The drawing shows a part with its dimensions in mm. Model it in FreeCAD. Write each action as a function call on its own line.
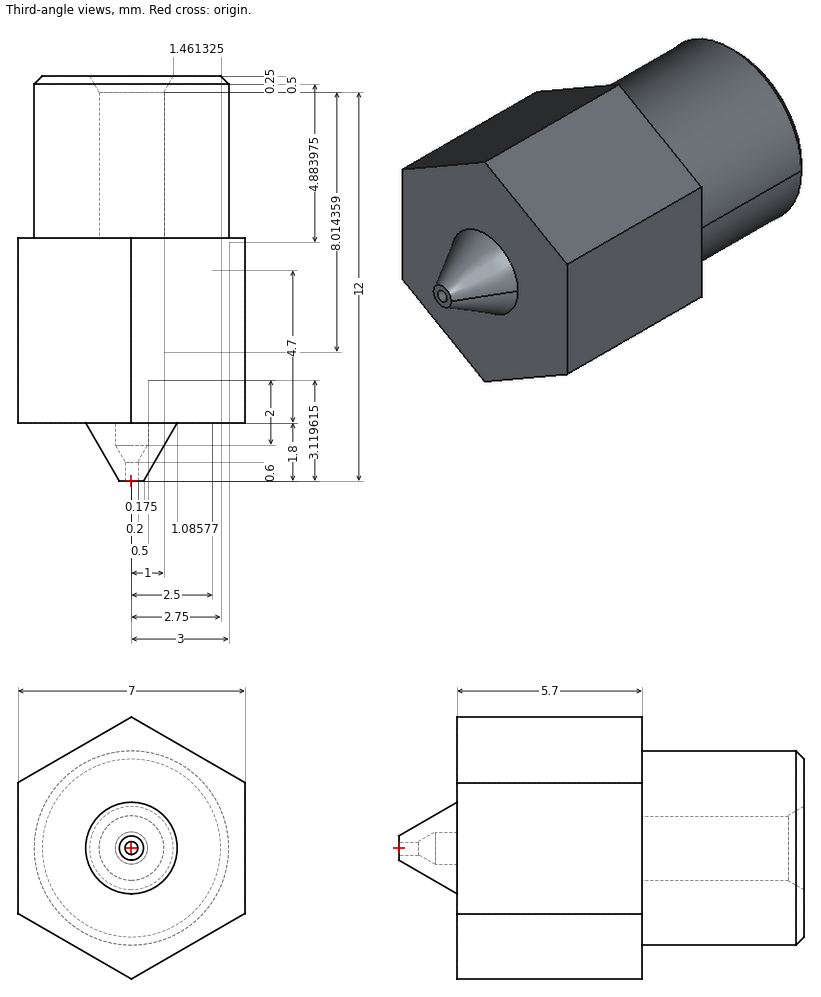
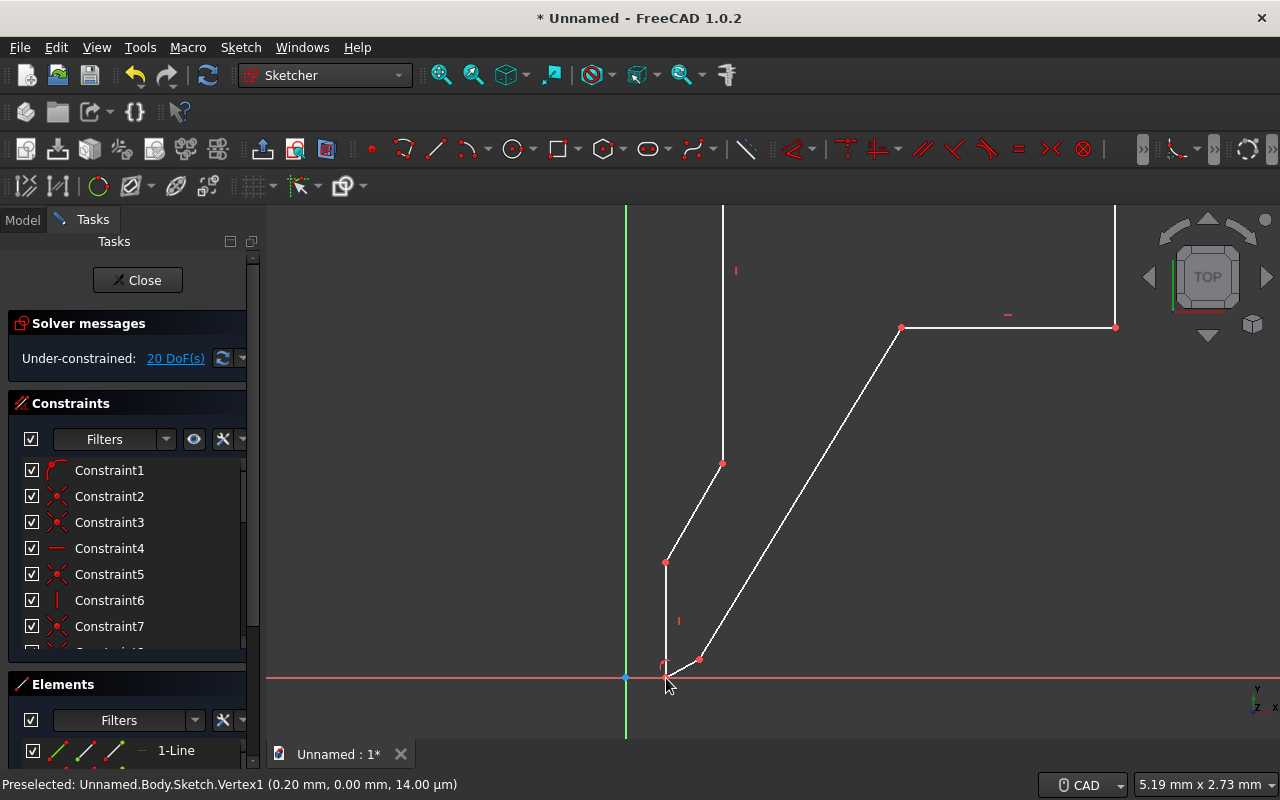
click(689, 665)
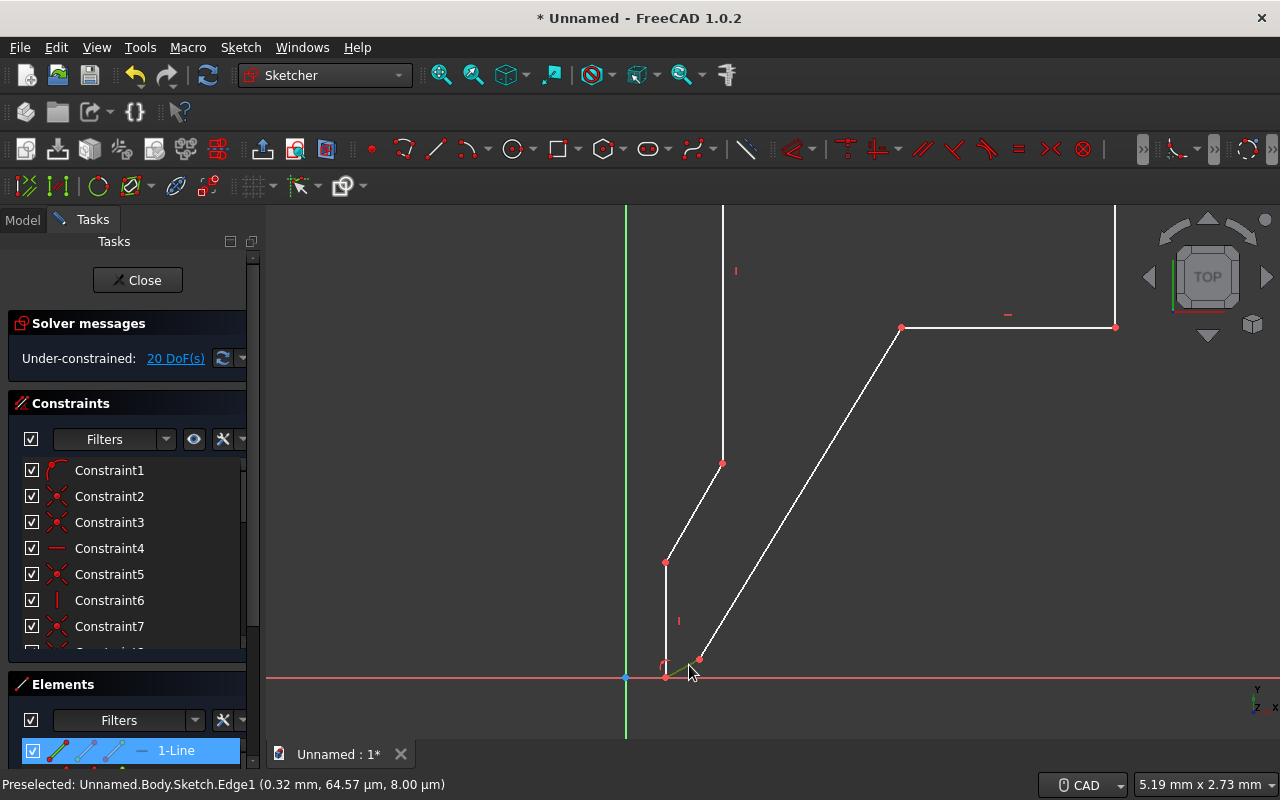
click(900, 150)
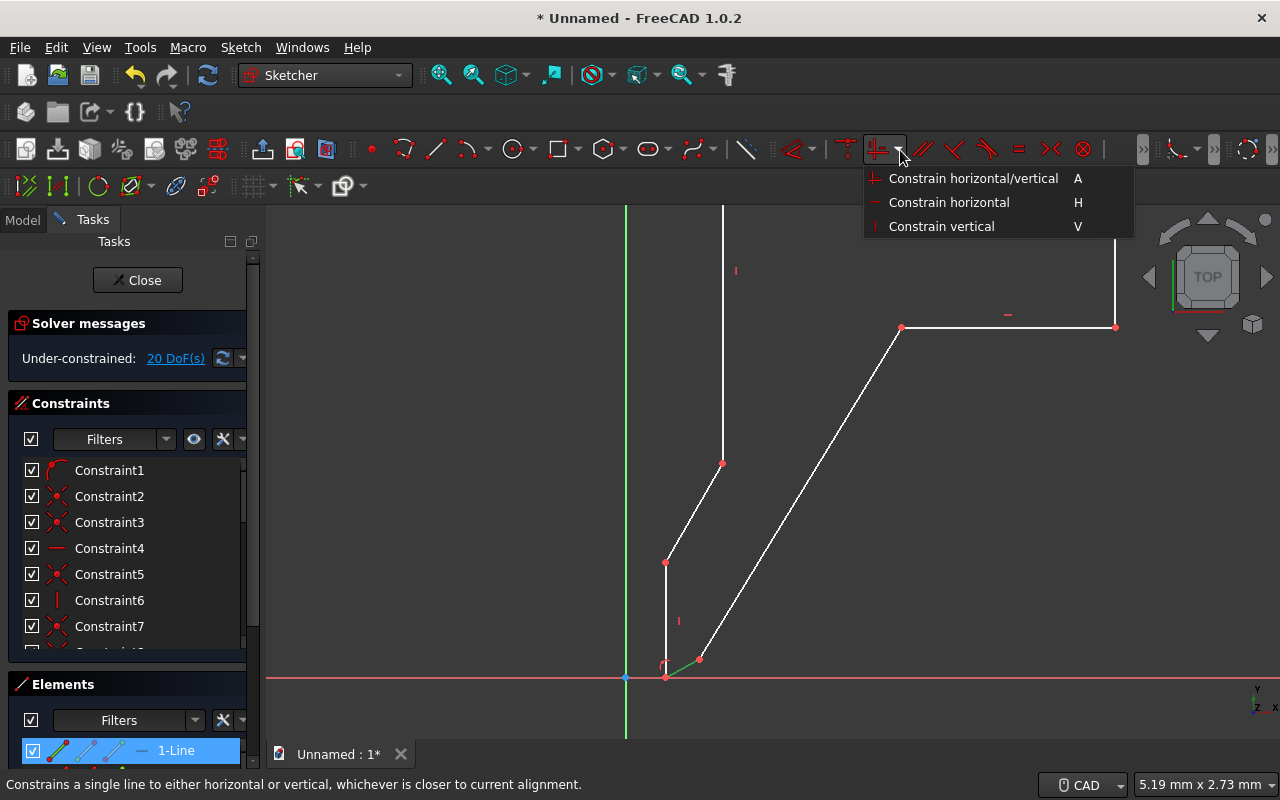
click(999, 202)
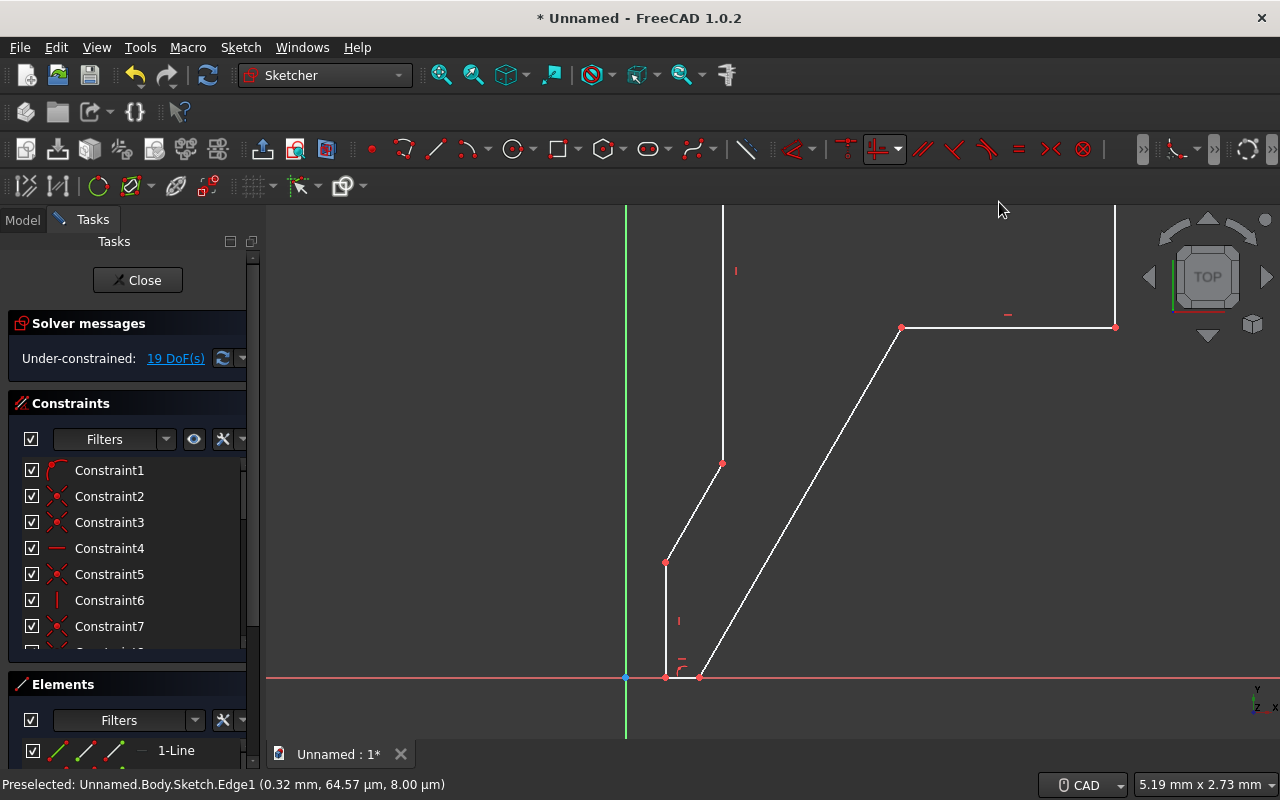
click(792, 150)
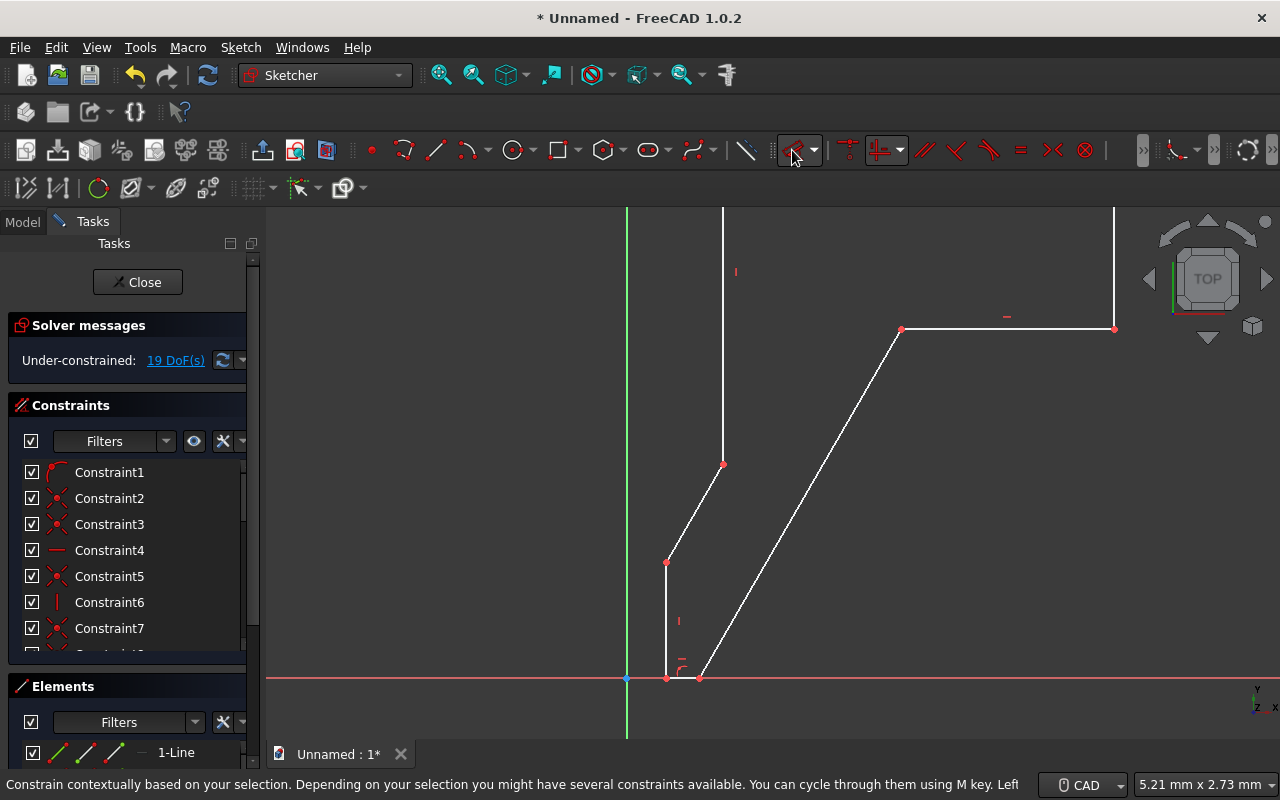
scroll(671, 631, down, 10)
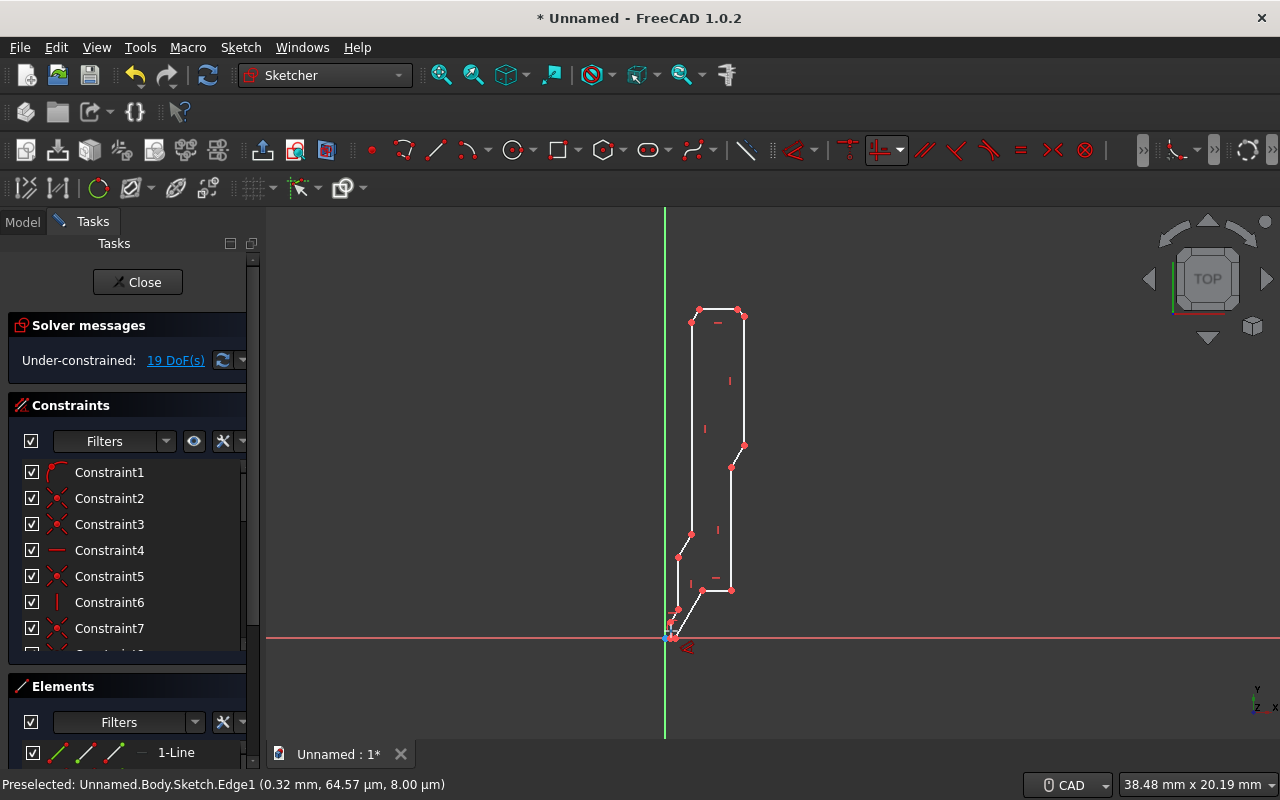
click(678, 594)
click(644, 583)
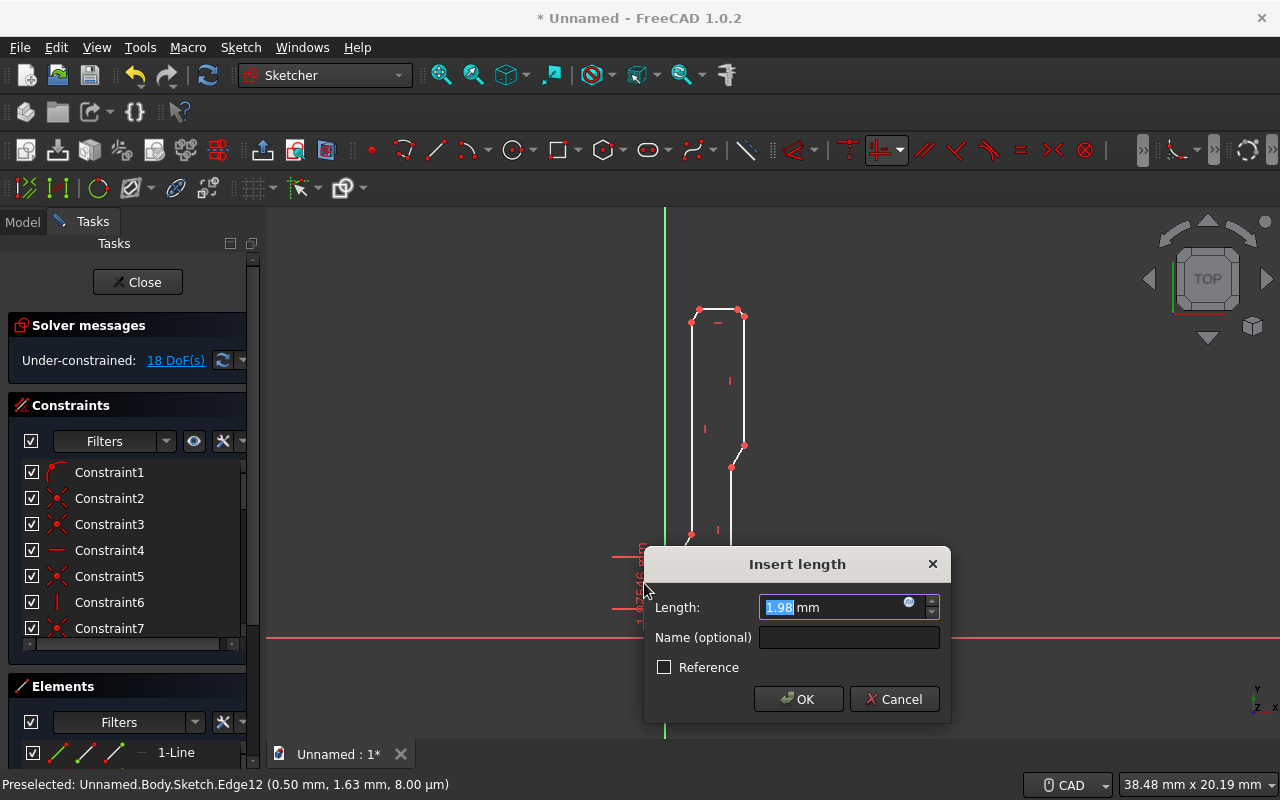
text(2)
key(Return)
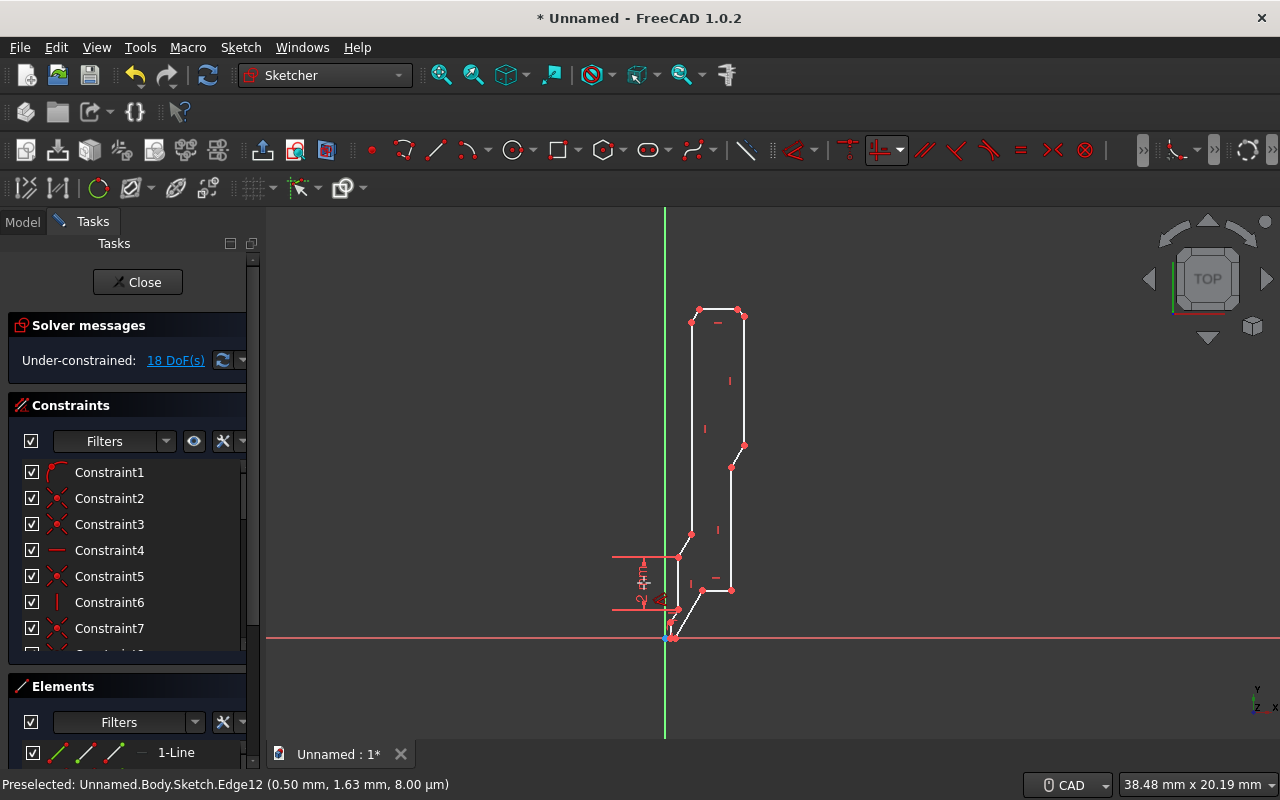
click(744, 445)
click(705, 672)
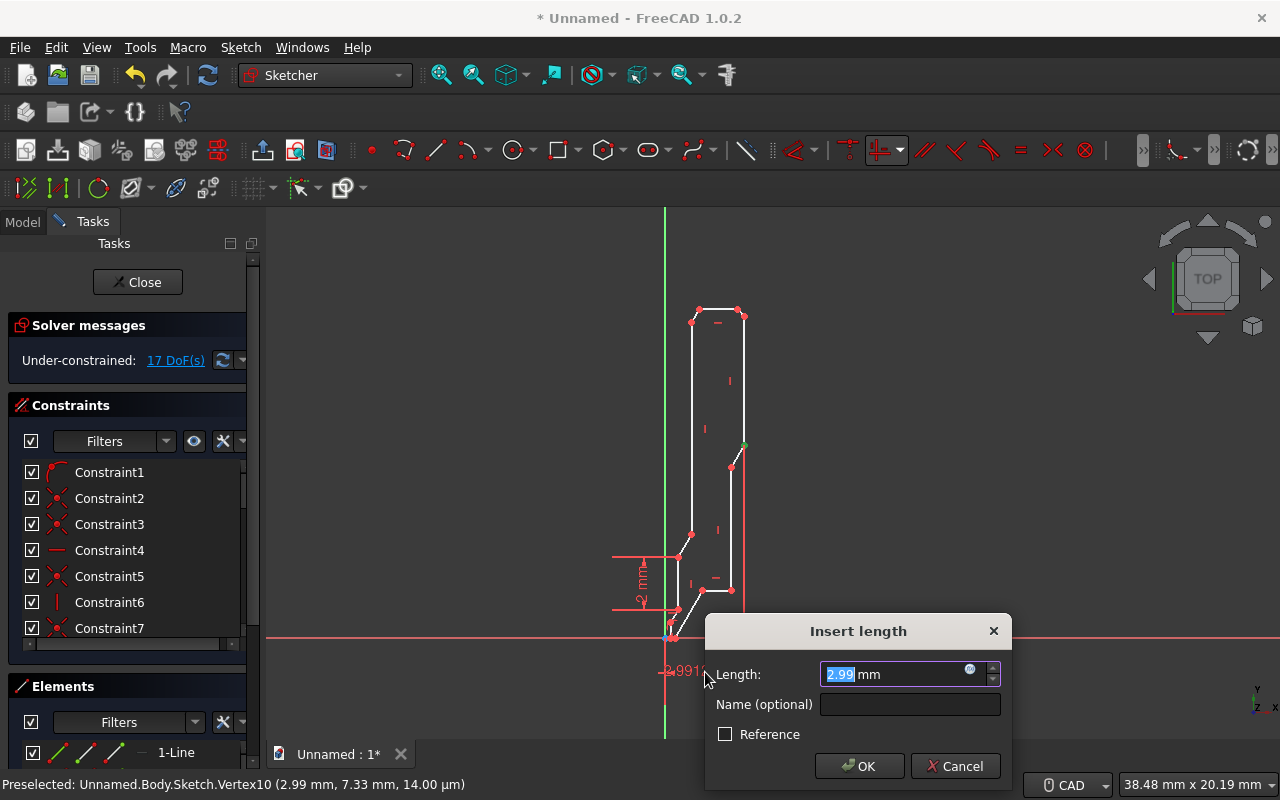
text(3)
key(Return)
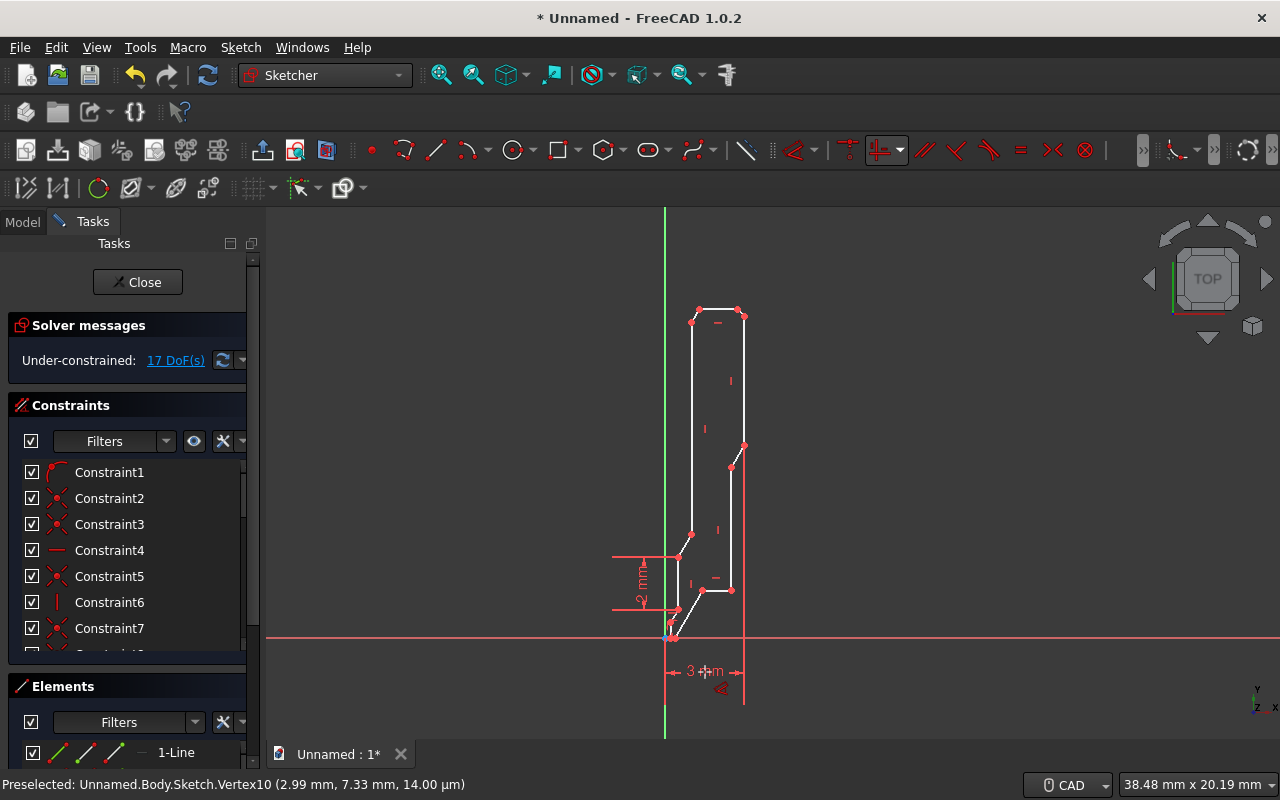
scroll(692, 322, up, 3)